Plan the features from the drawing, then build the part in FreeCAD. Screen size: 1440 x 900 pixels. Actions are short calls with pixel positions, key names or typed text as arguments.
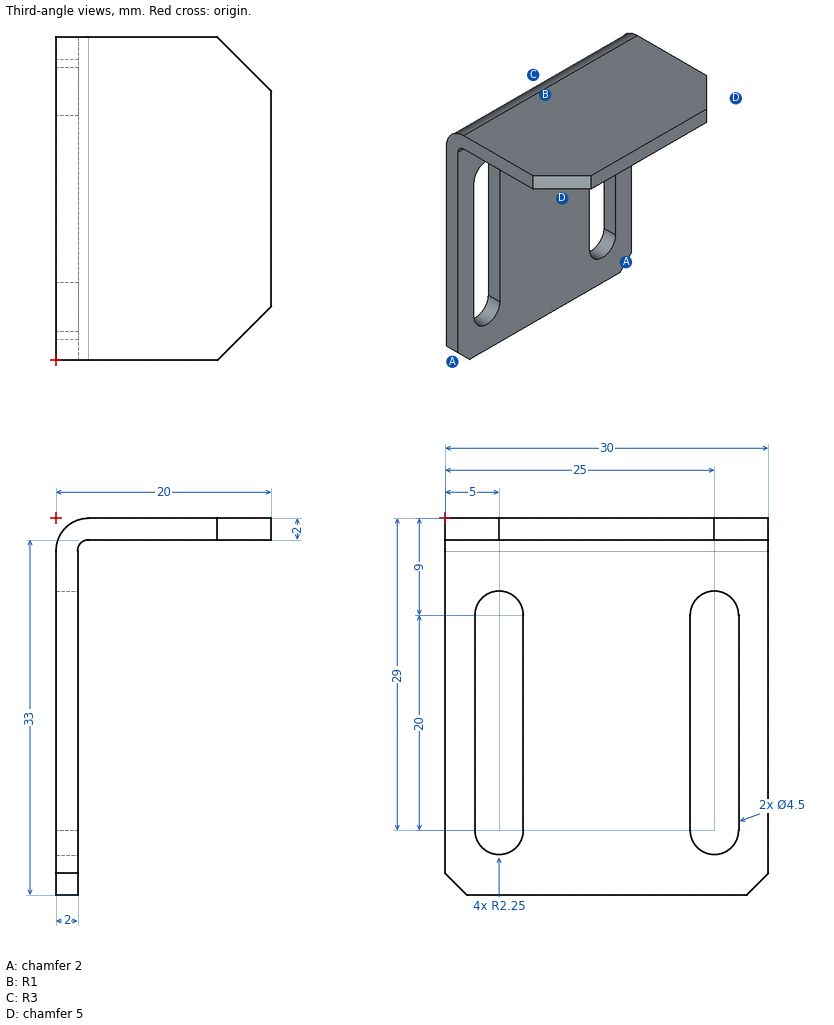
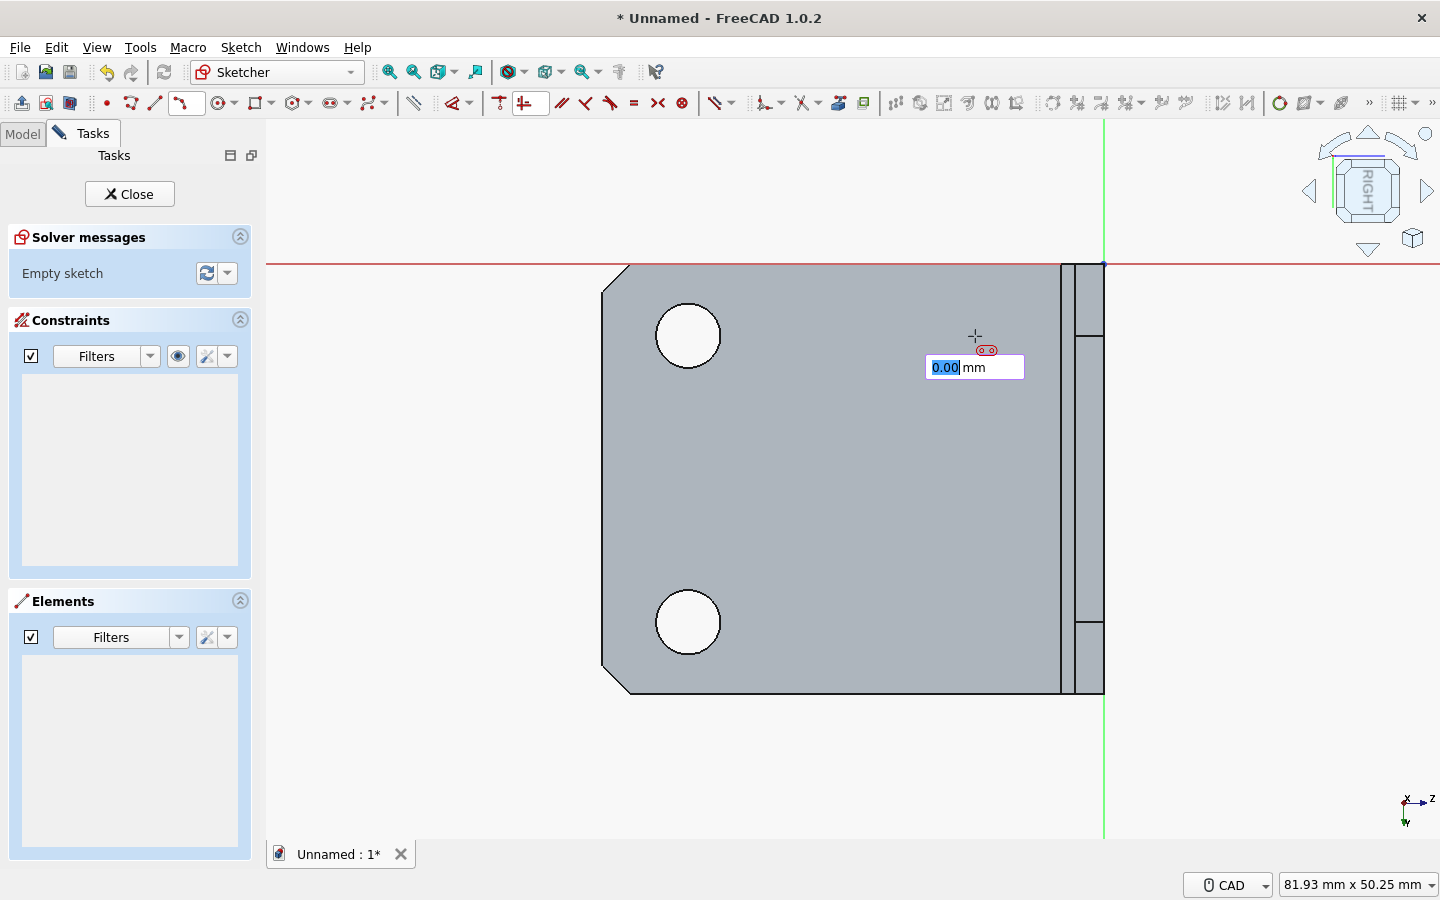
click(832, 303)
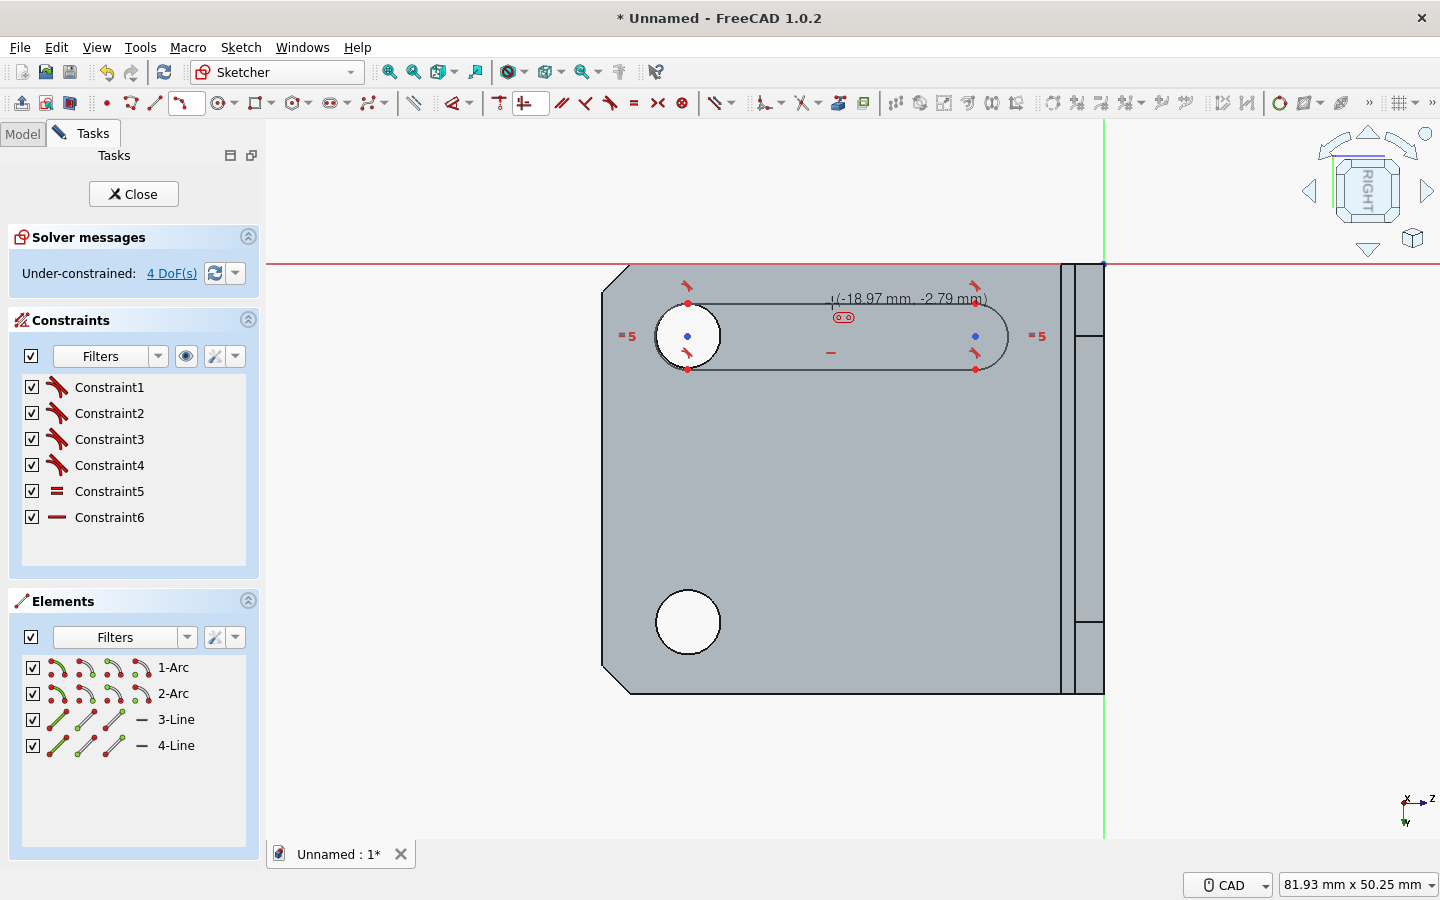
click(688, 622)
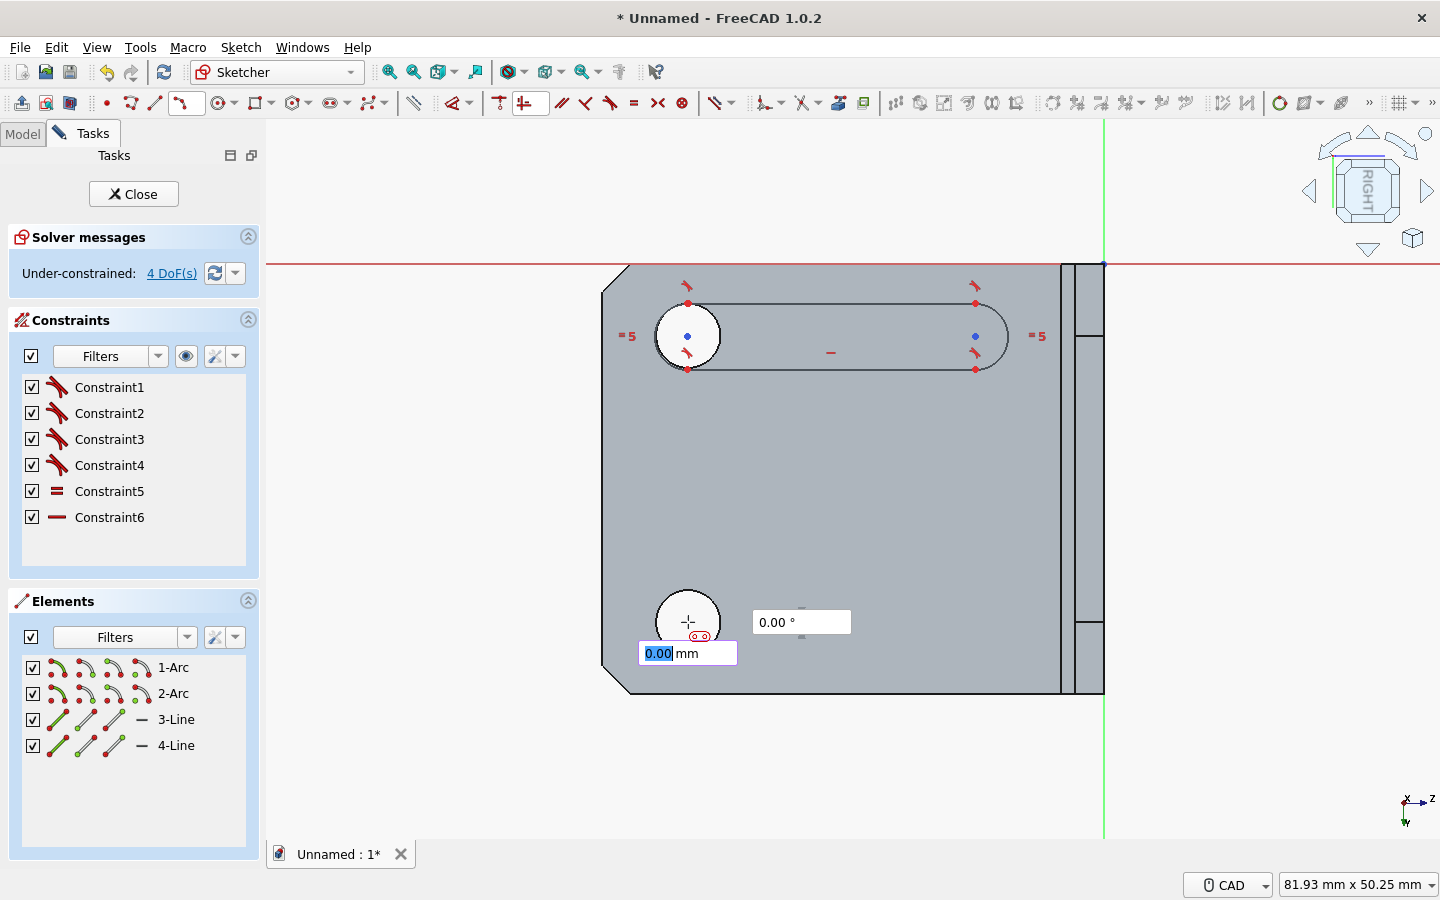
click(975, 622)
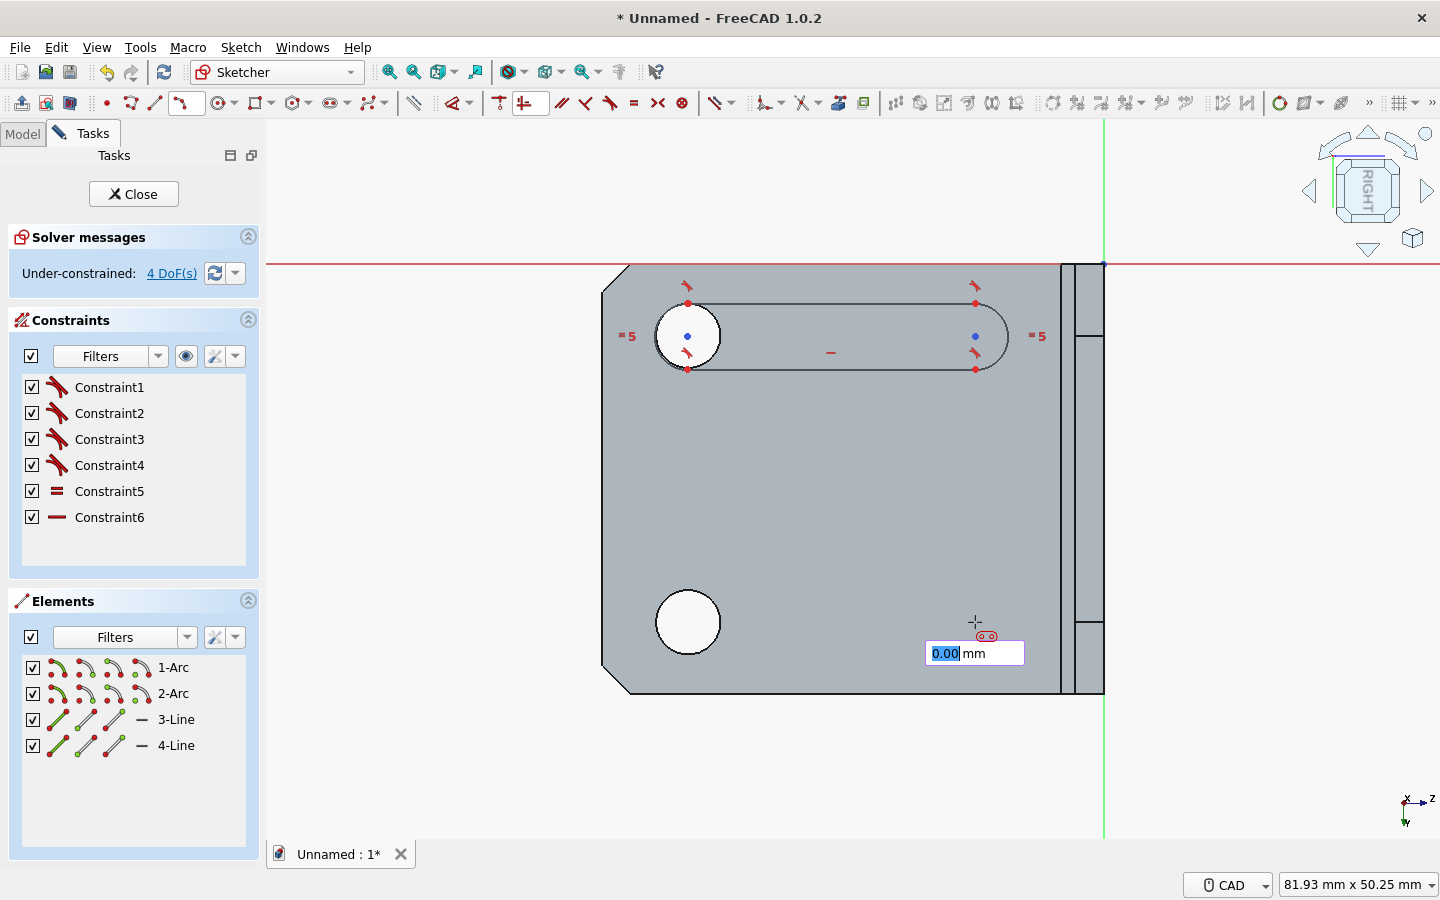
click(832, 655)
key(Escape)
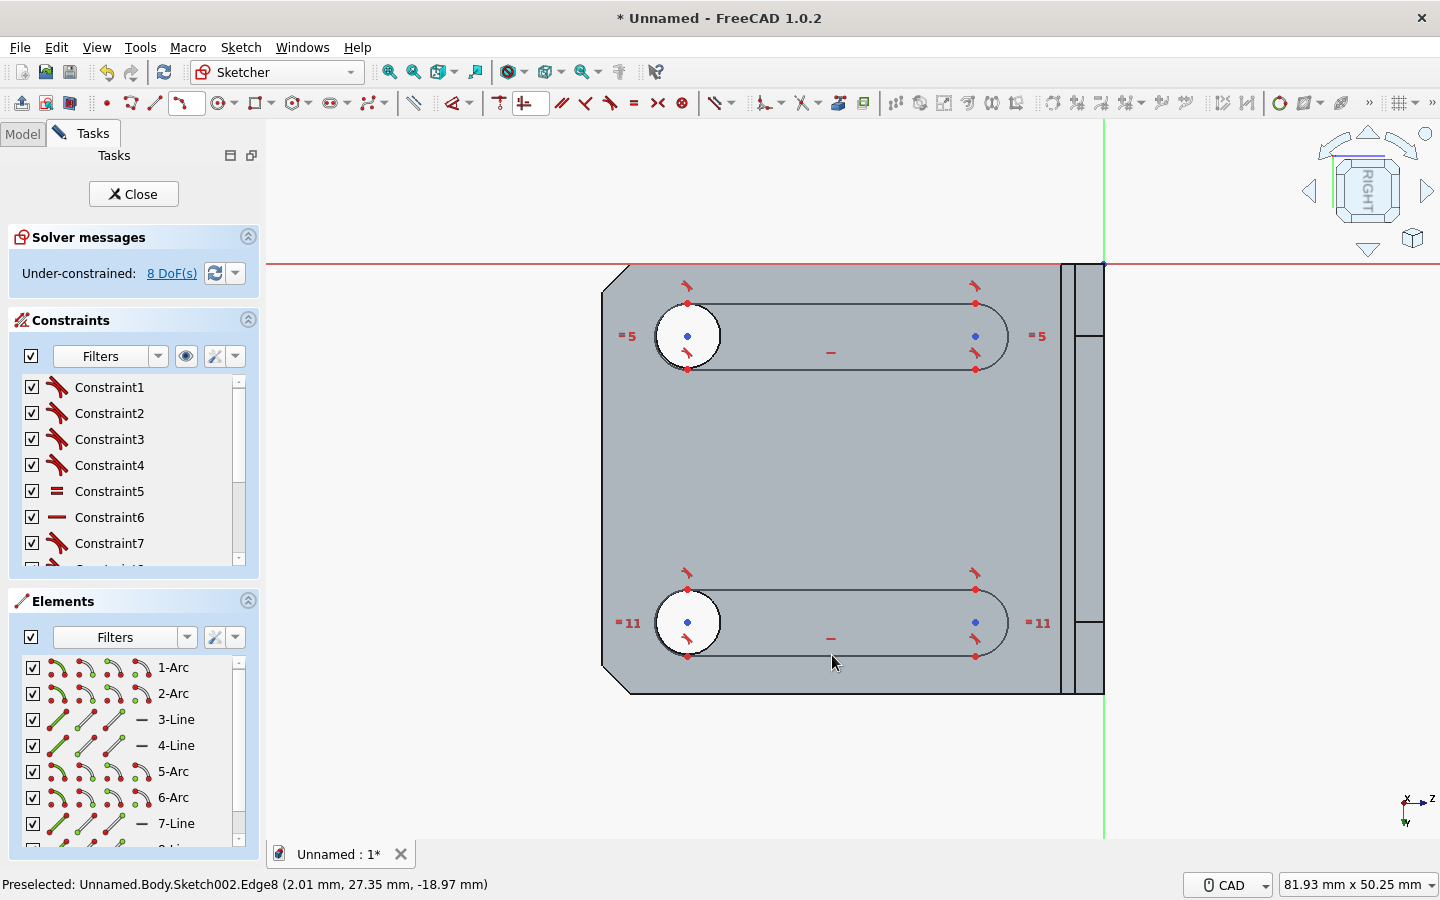
click(661, 318)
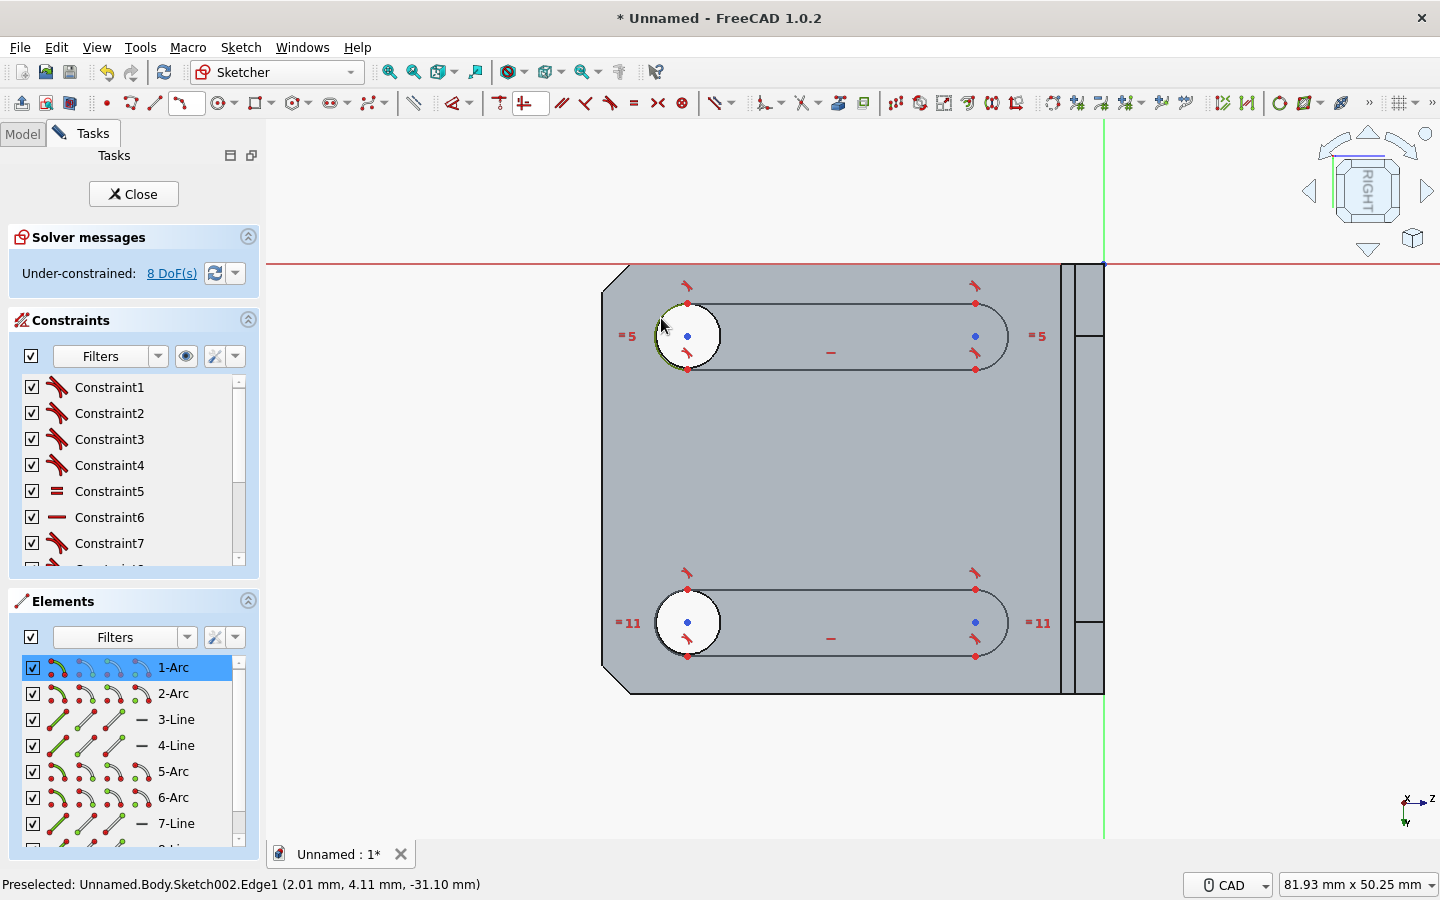
click(661, 604)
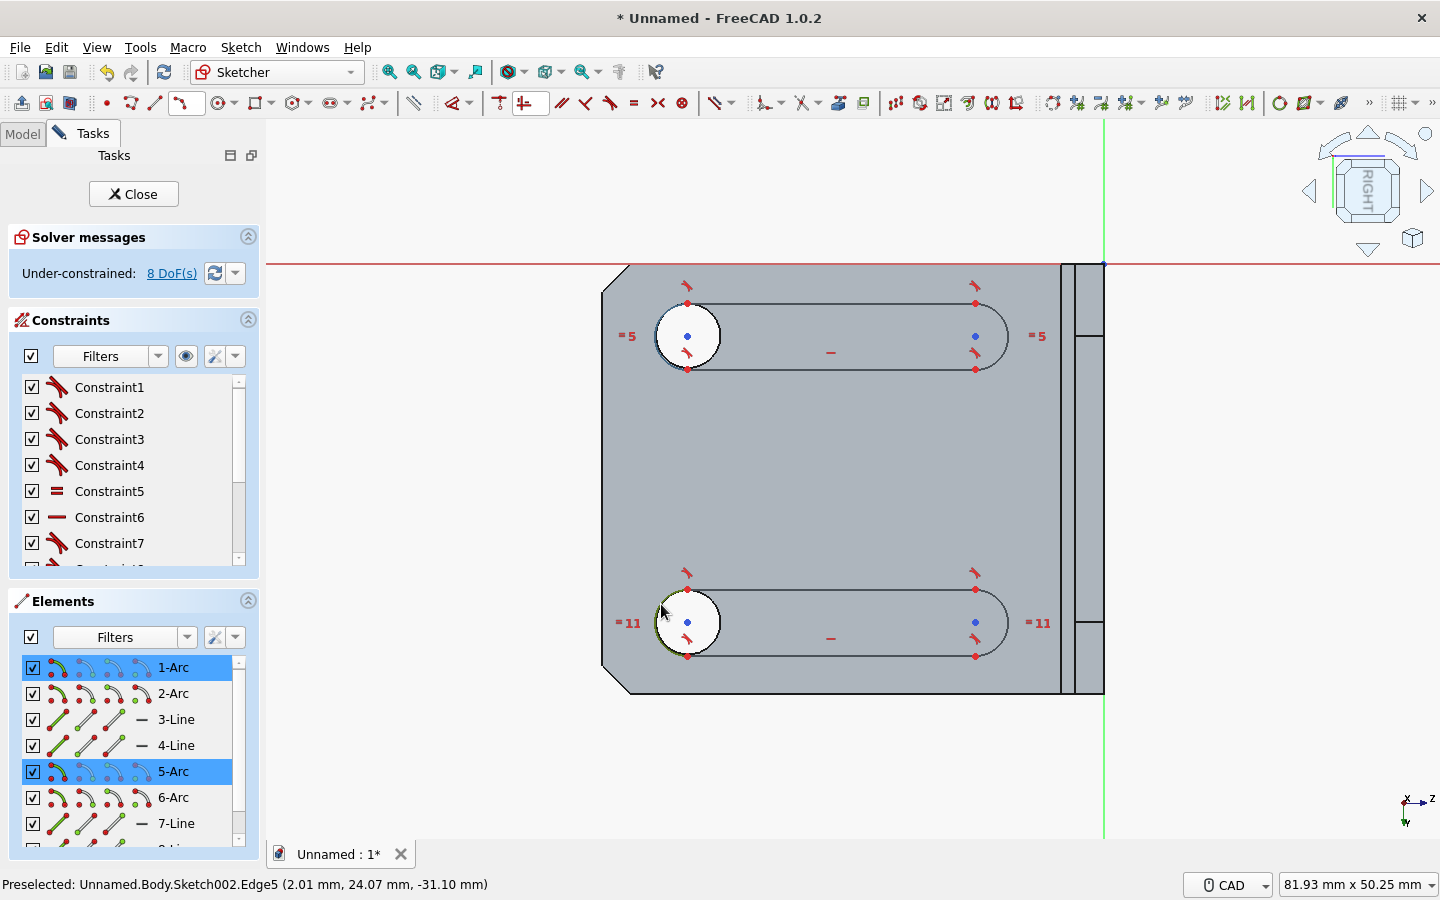
click(634, 104)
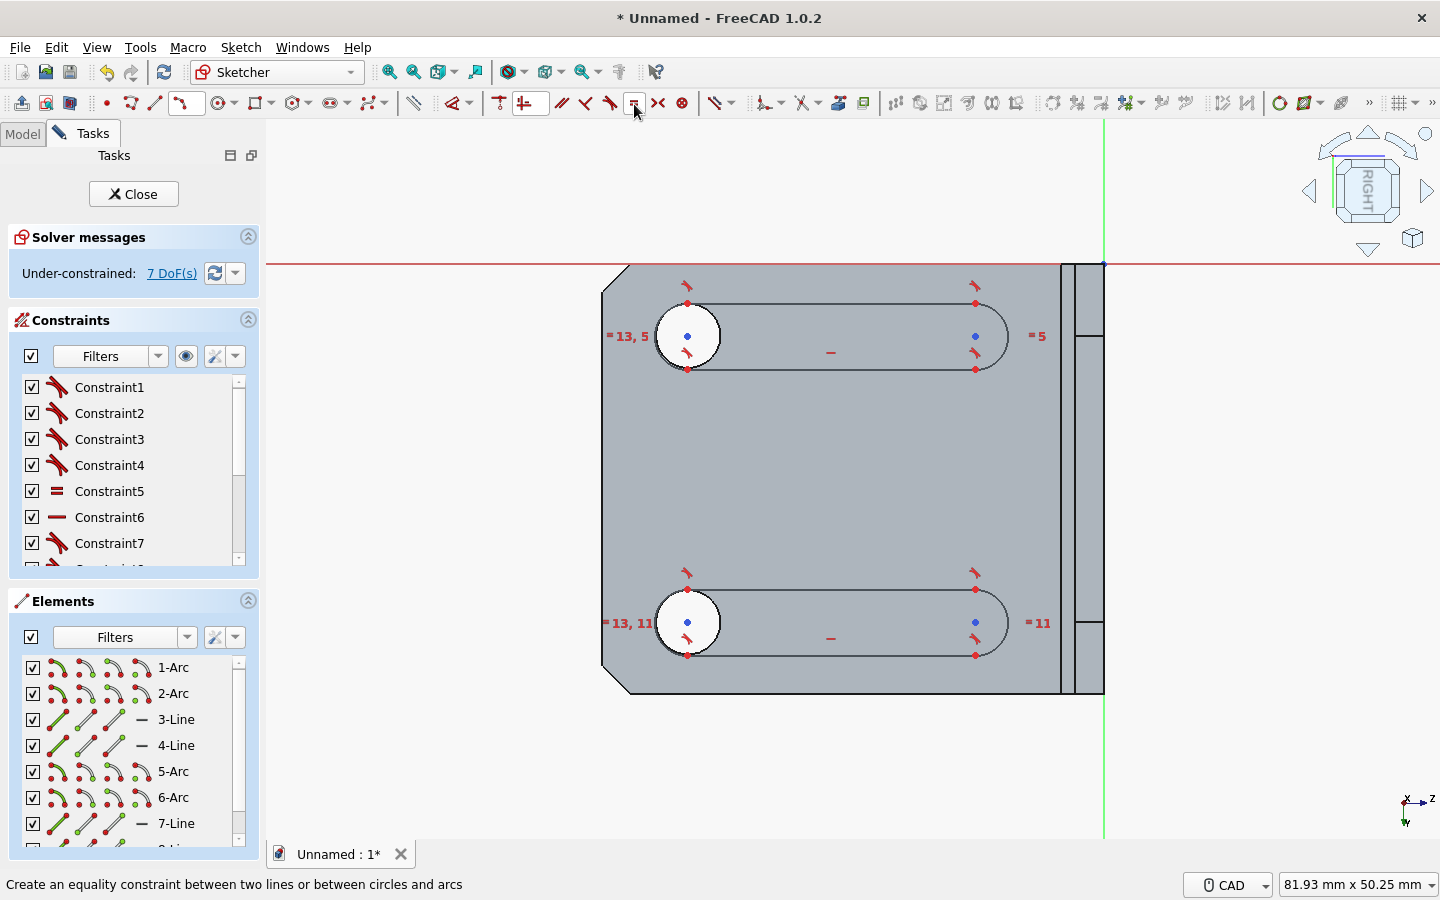
click(452, 104)